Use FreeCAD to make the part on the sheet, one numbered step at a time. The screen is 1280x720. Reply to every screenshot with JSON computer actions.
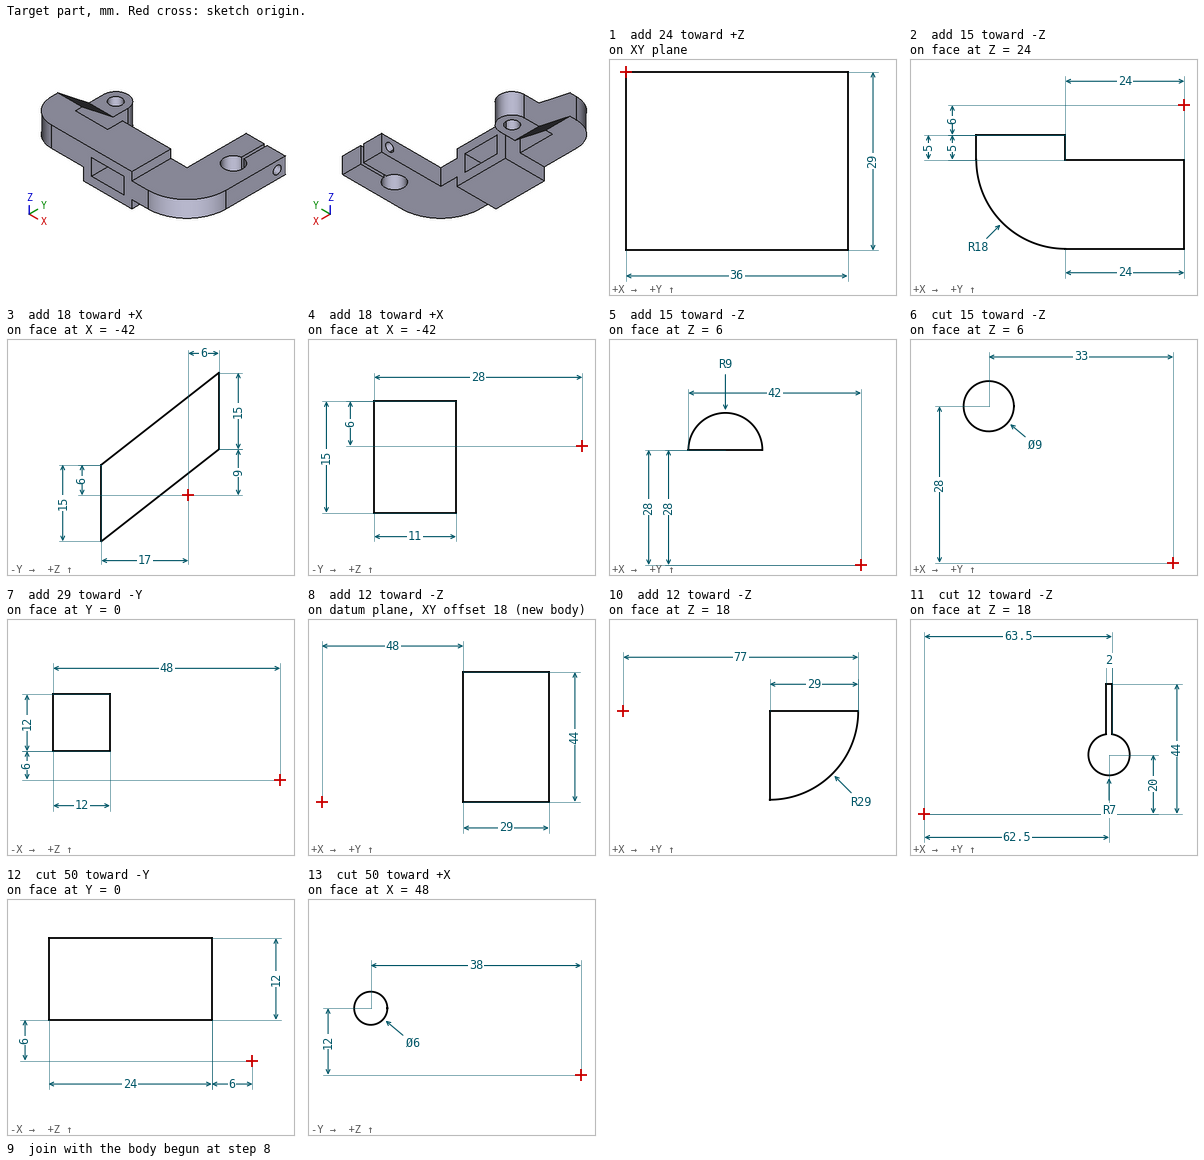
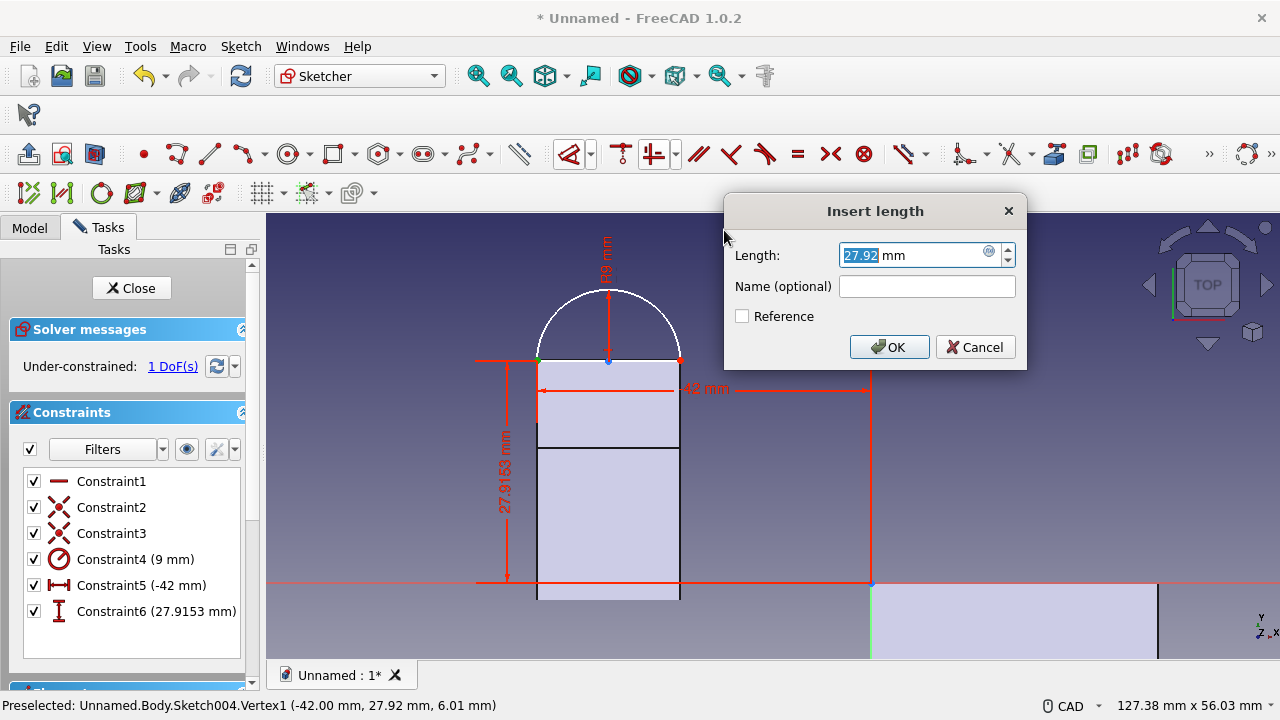
{"action": "type", "text": "28"}
{"action": "key", "text": "Return"}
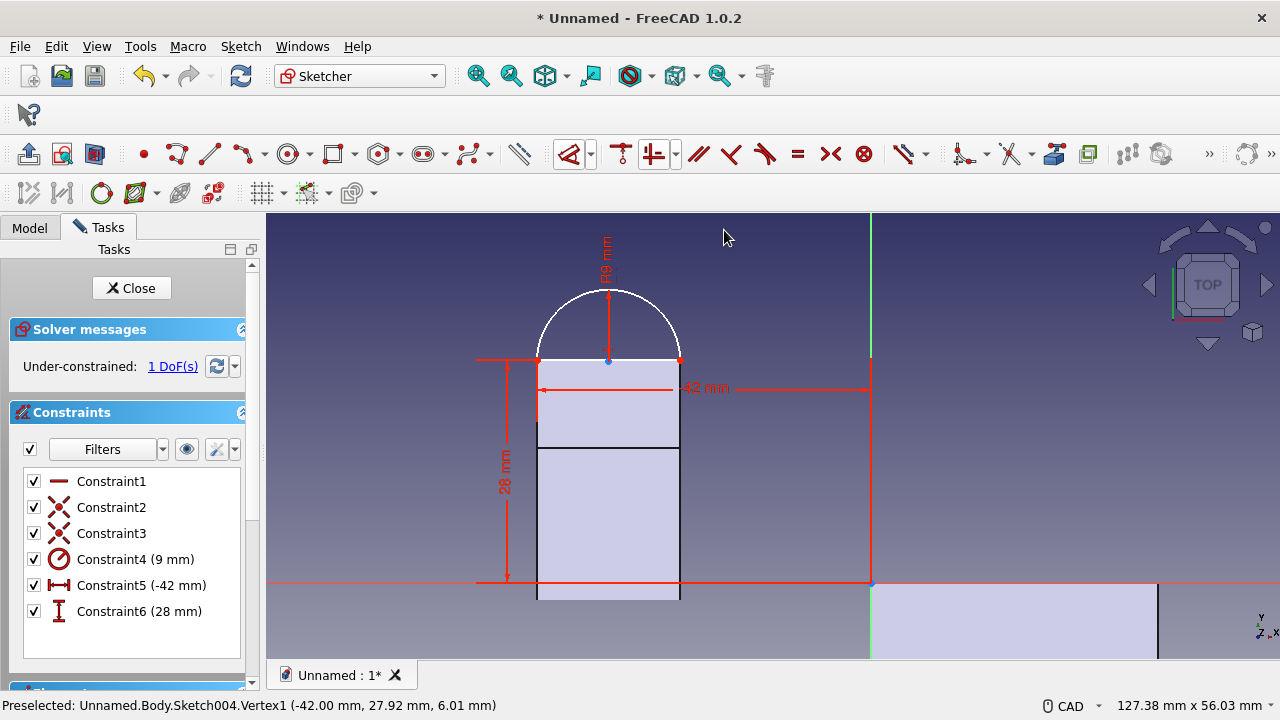
{"action": "left_click", "coordinate": [609, 362]}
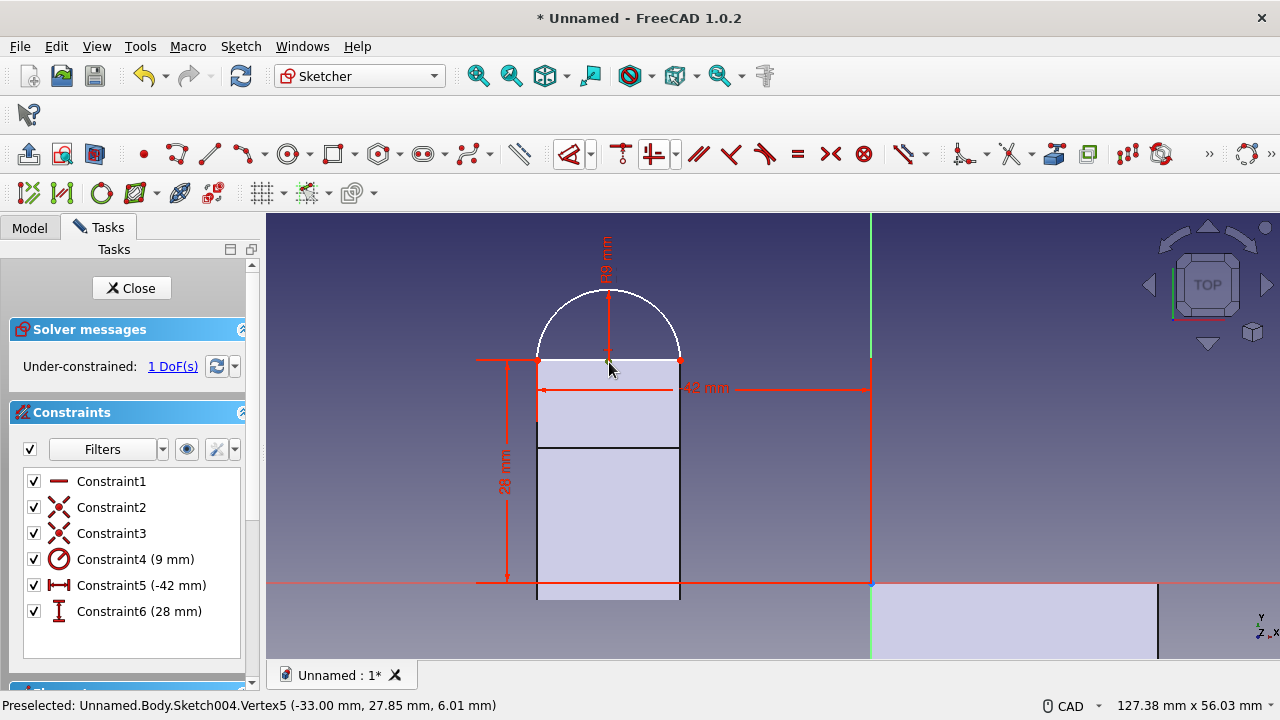
{"action": "key", "text": "i"}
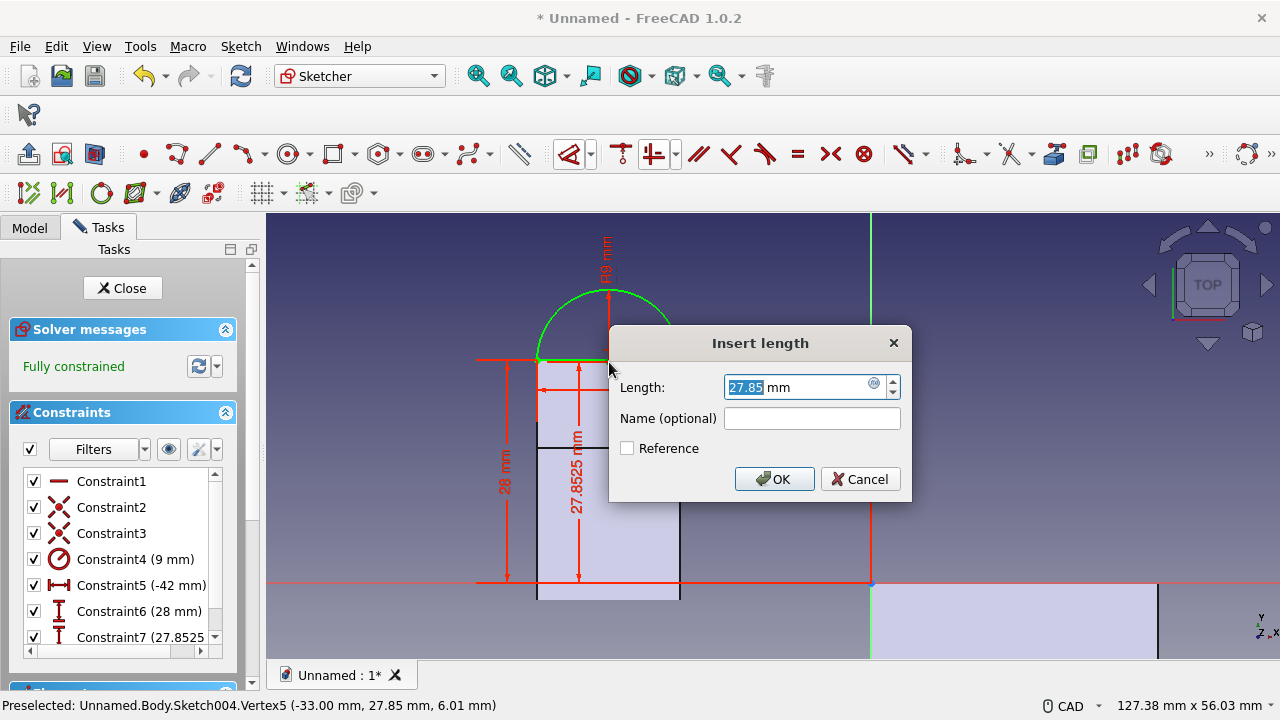
{"action": "type", "text": "28"}
{"action": "key", "text": "Return"}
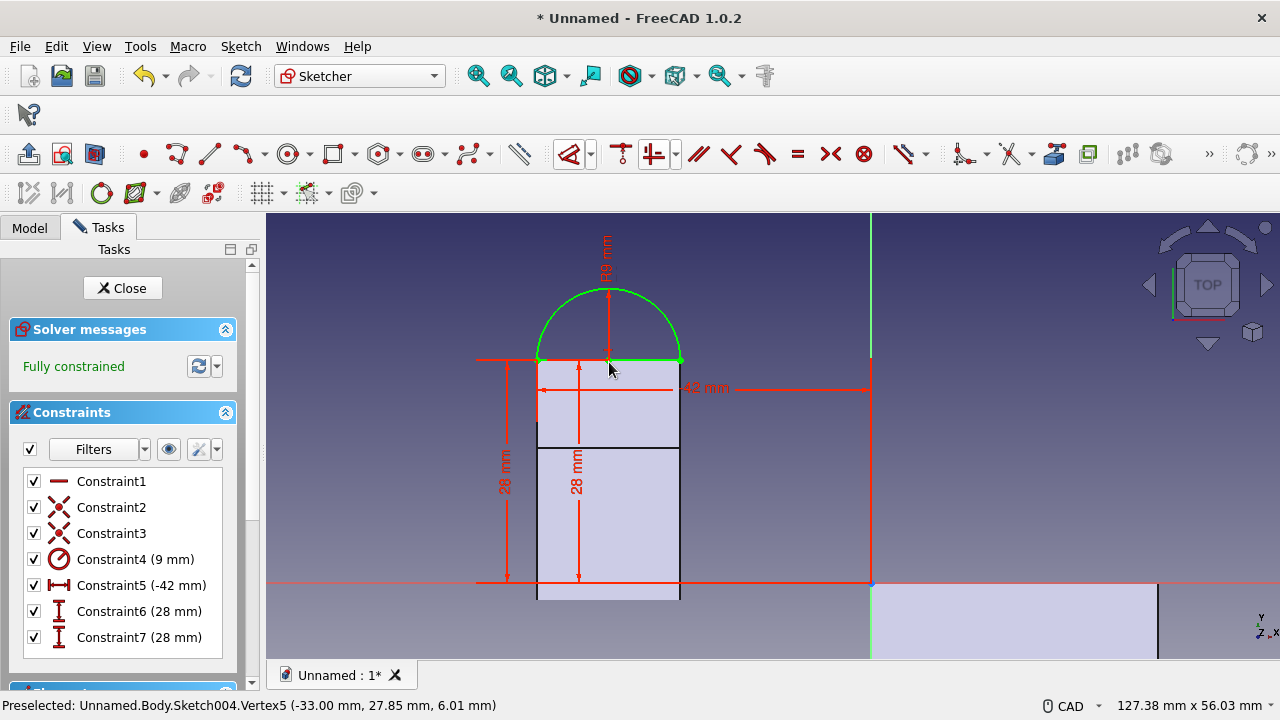
{"action": "left_click", "coordinate": [123, 288]}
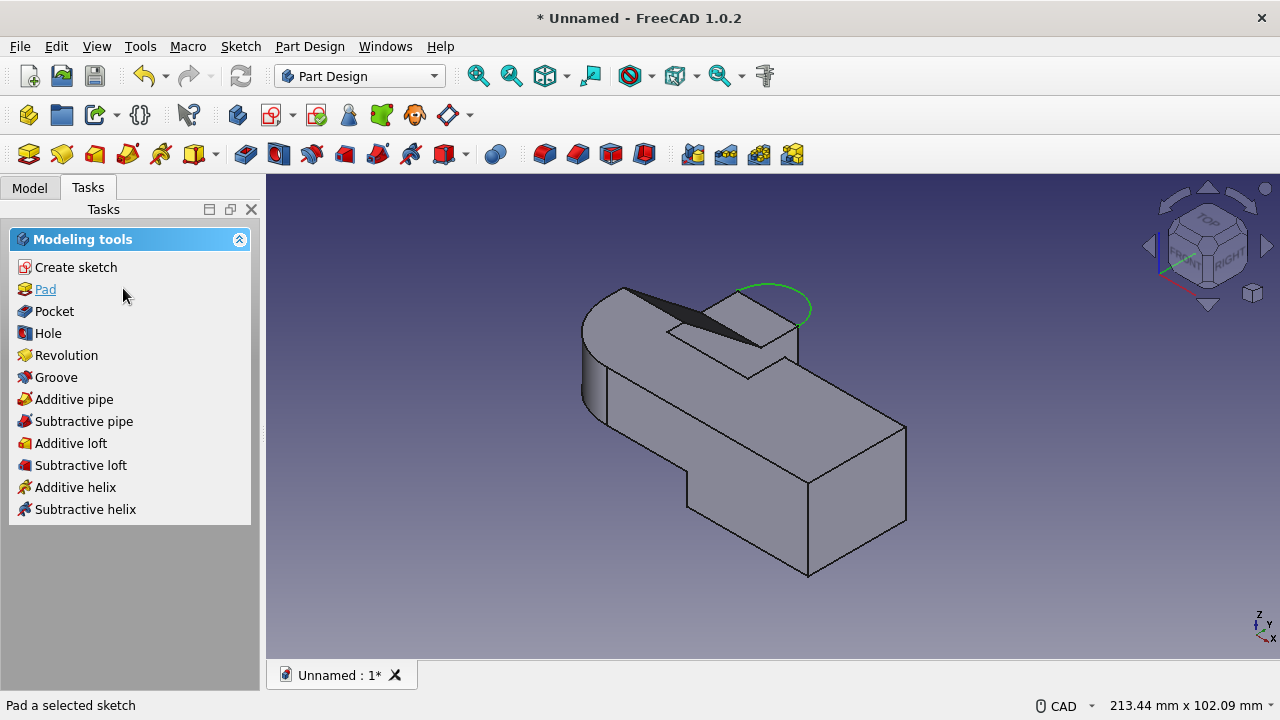
{"action": "left_click", "coordinate": [29, 154]}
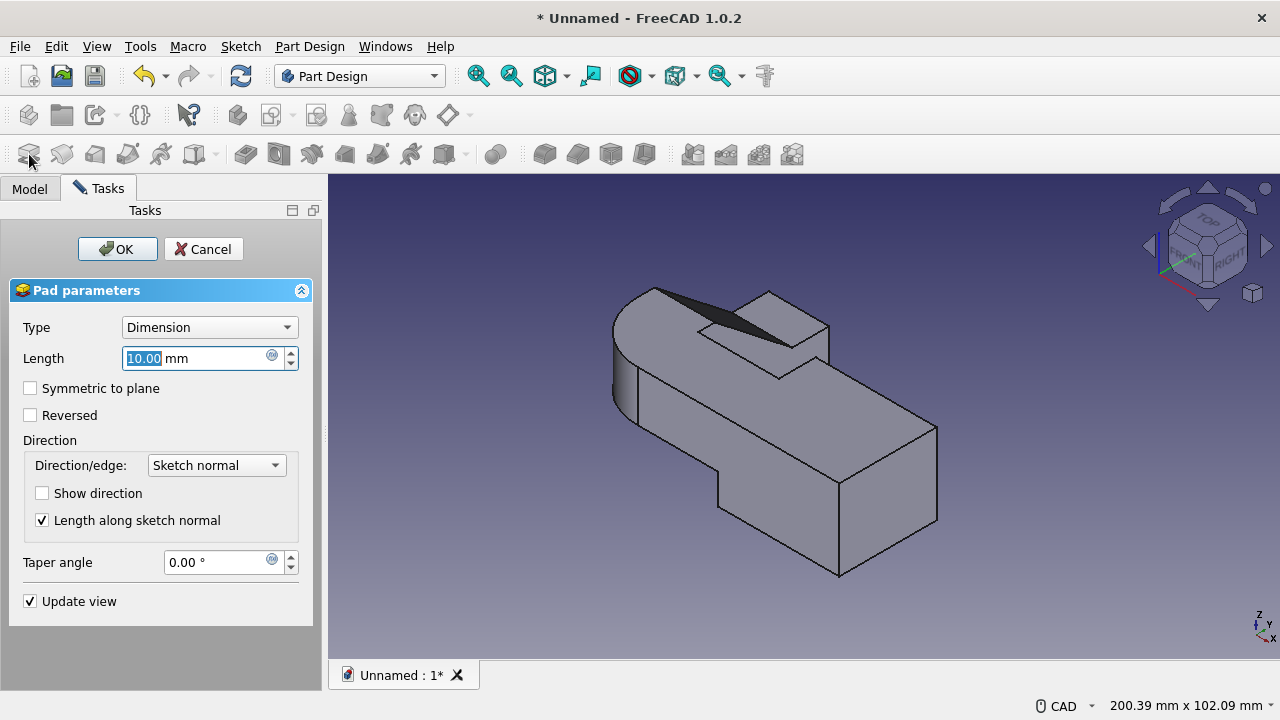
{"action": "type", "text": "15"}
{"action": "key", "text": "Tab"}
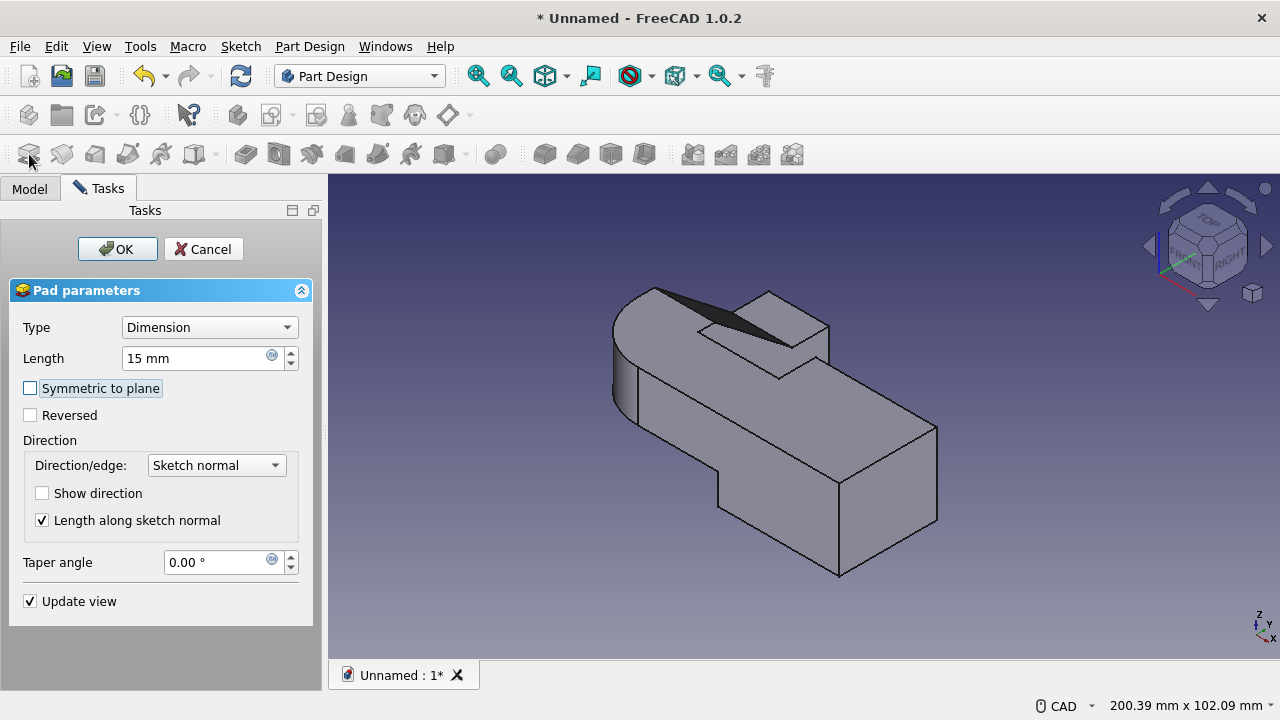
{"action": "left_click", "coordinate": [31, 415]}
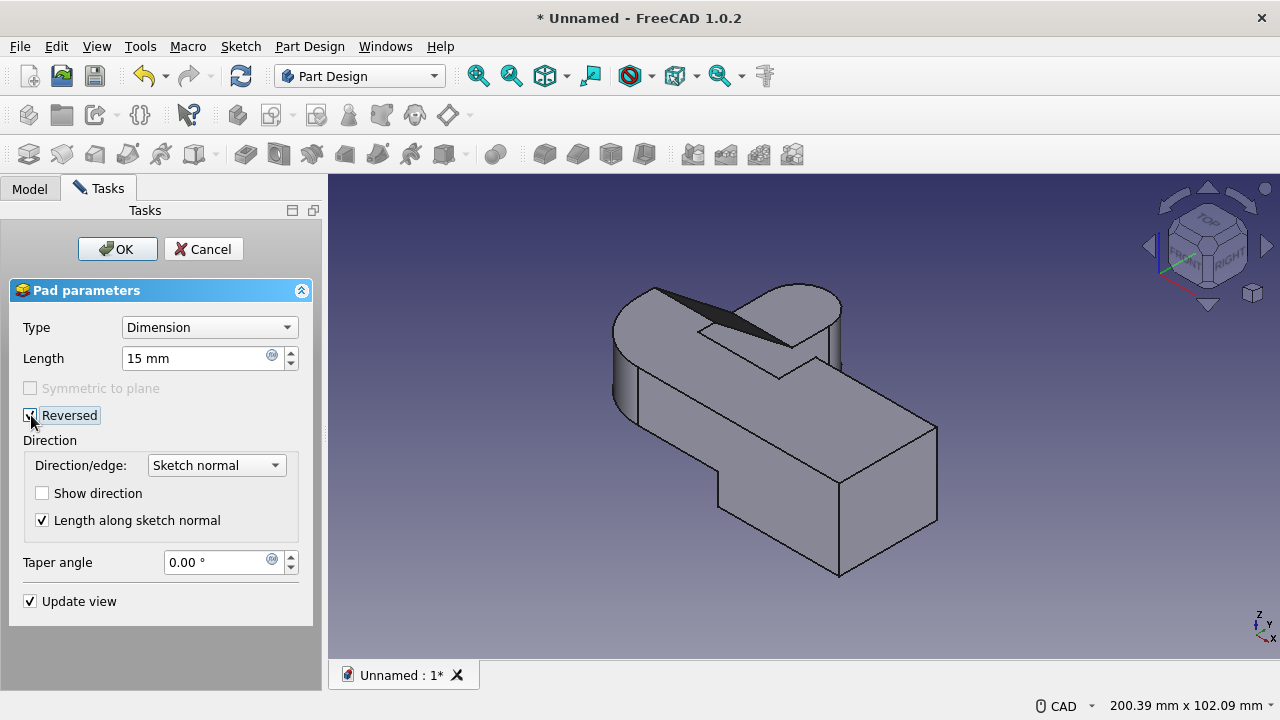
{"action": "left_click", "coordinate": [118, 249]}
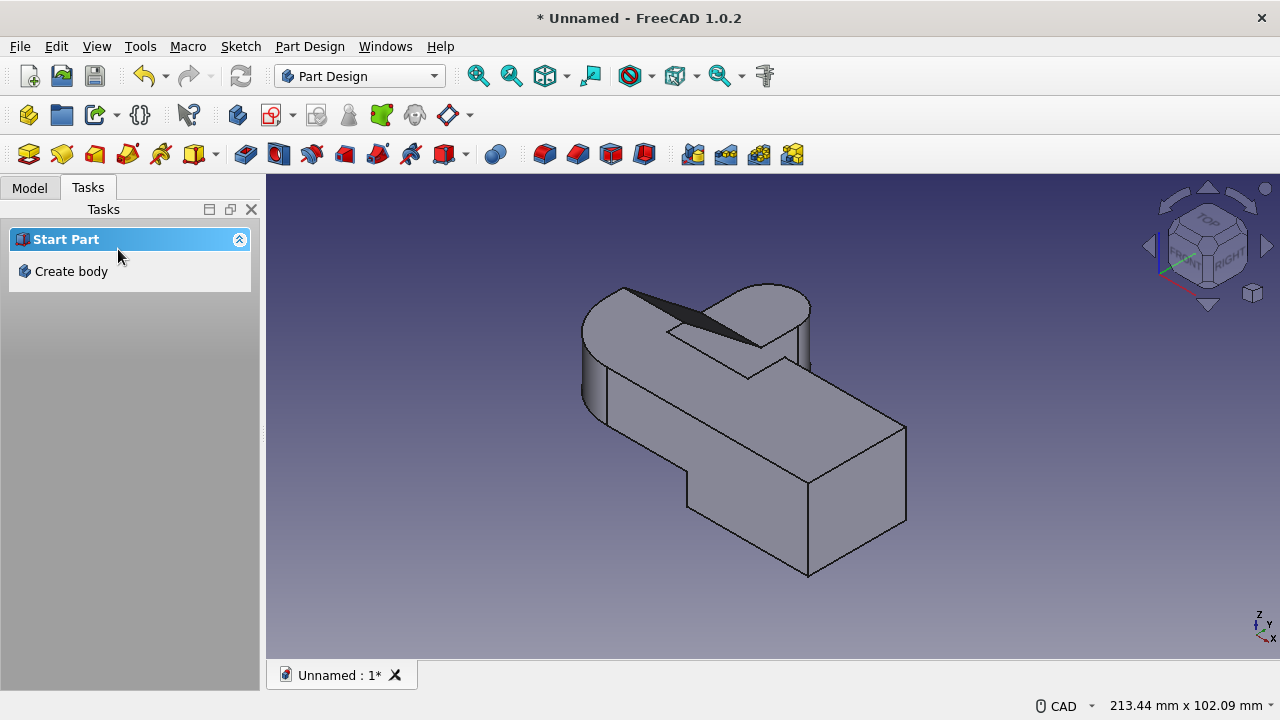
{"action": "left_click", "coordinate": [765, 310]}